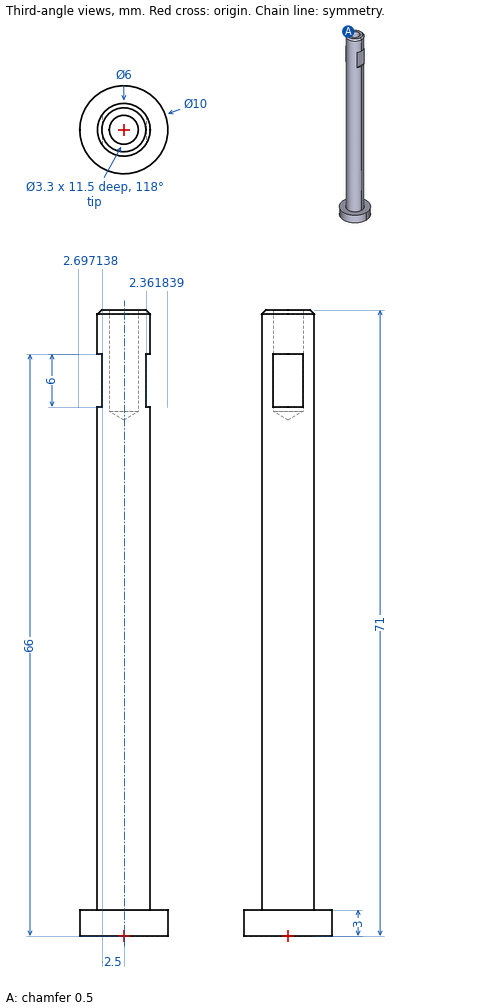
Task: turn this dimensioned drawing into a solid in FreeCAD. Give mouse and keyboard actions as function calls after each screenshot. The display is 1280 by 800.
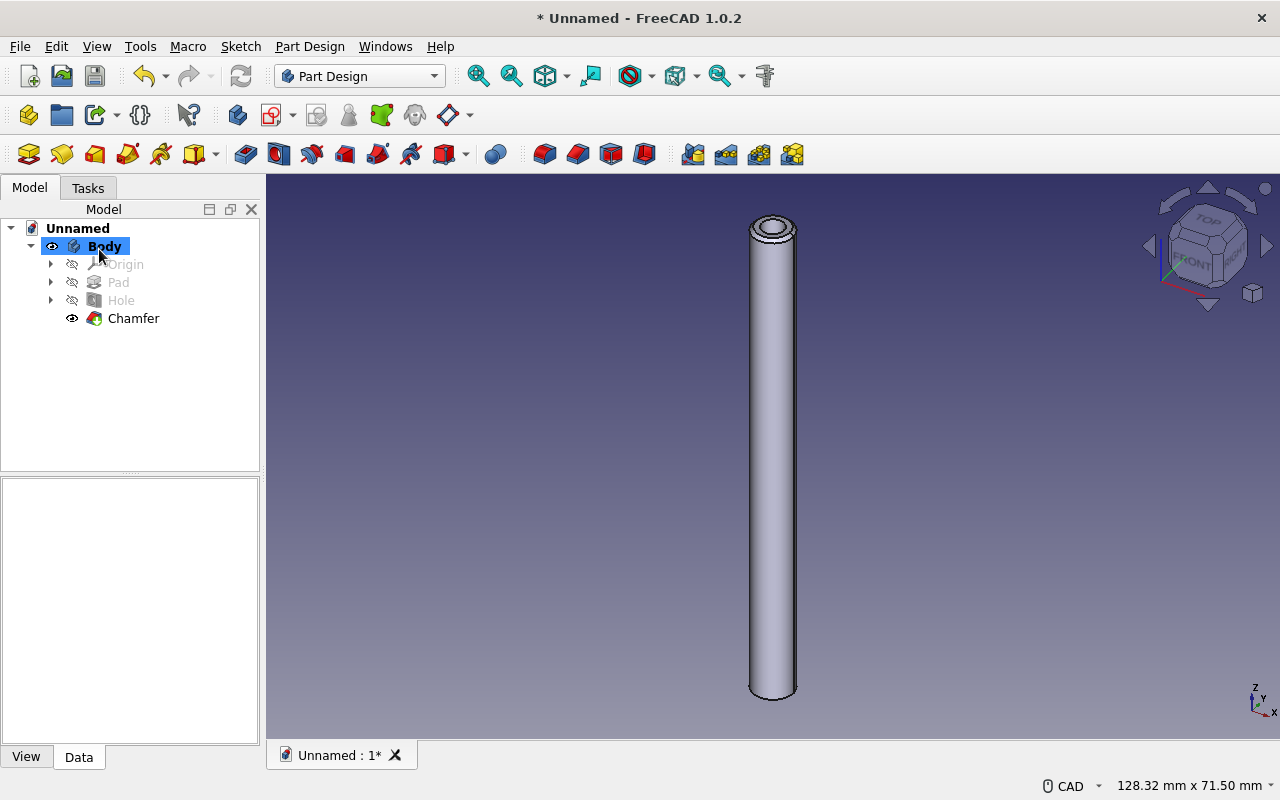
click(270, 116)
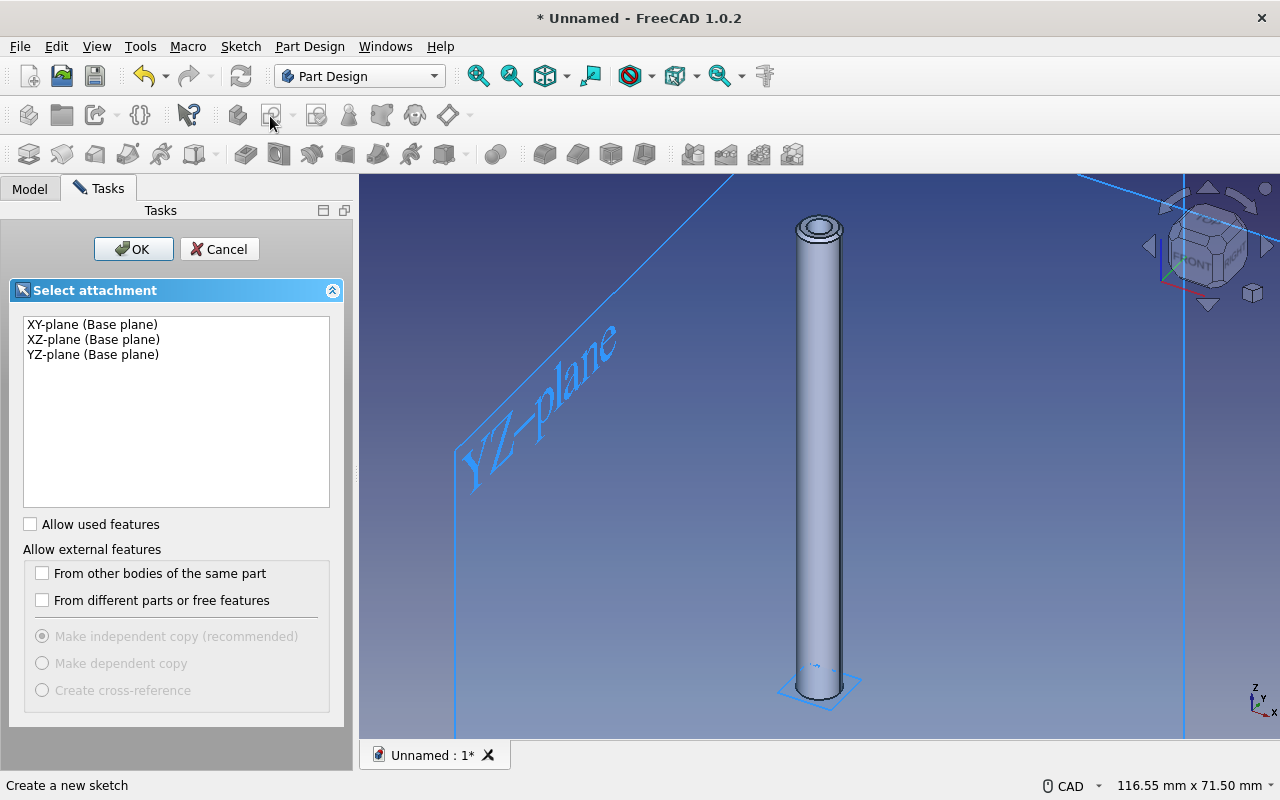
click(84, 340)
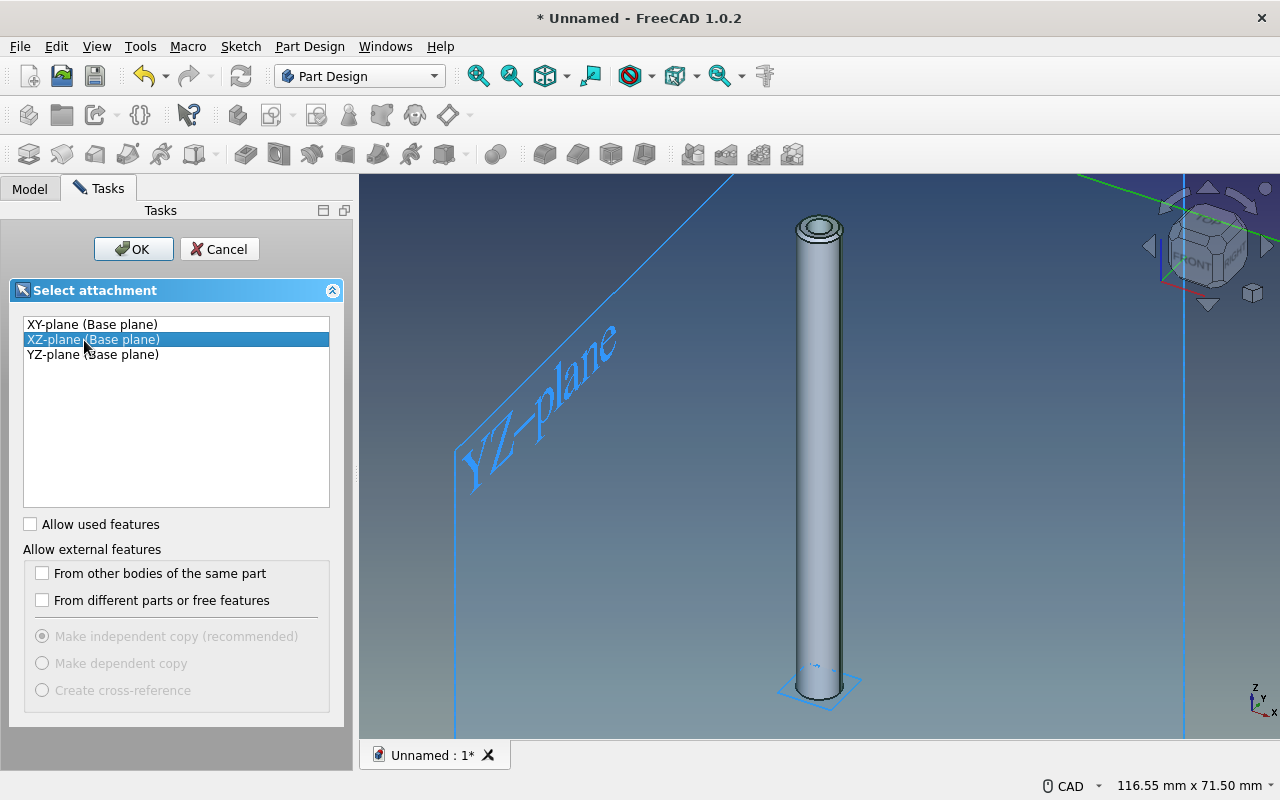
click(134, 249)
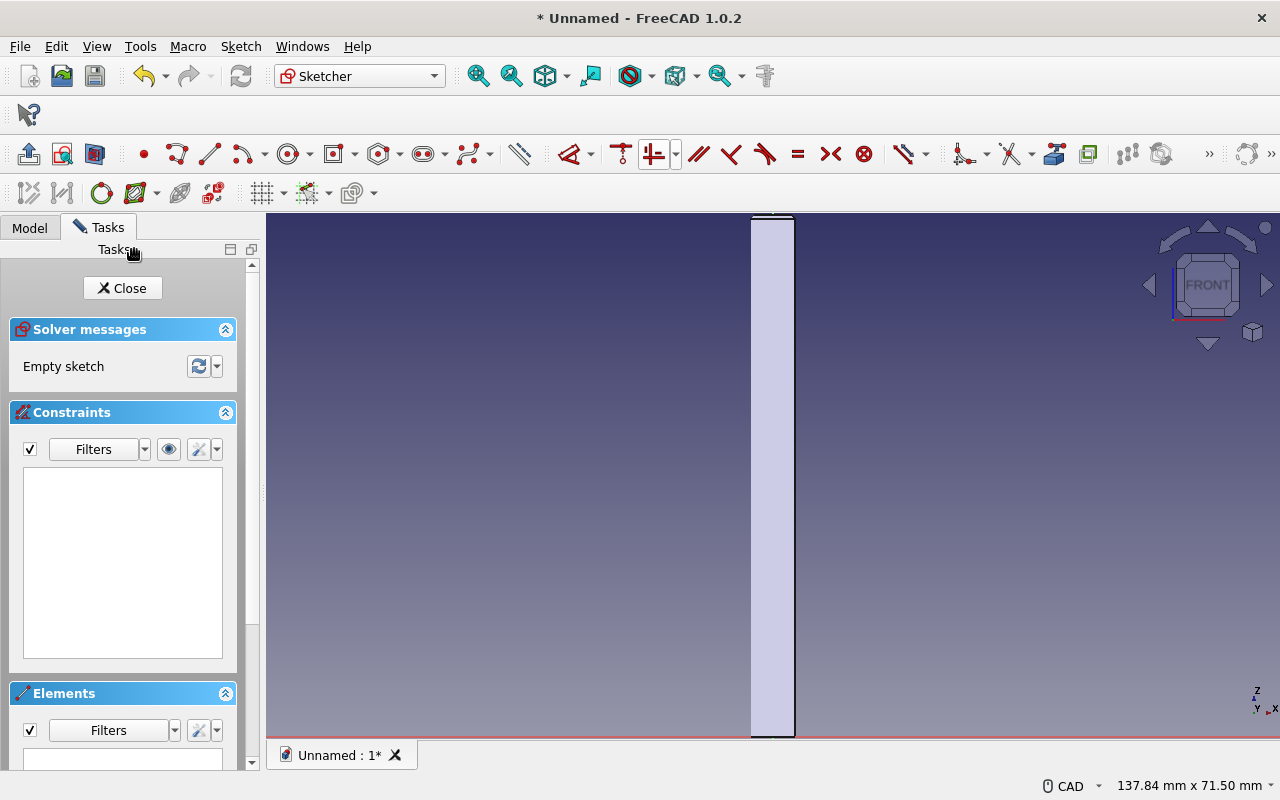
key(q)
key(s)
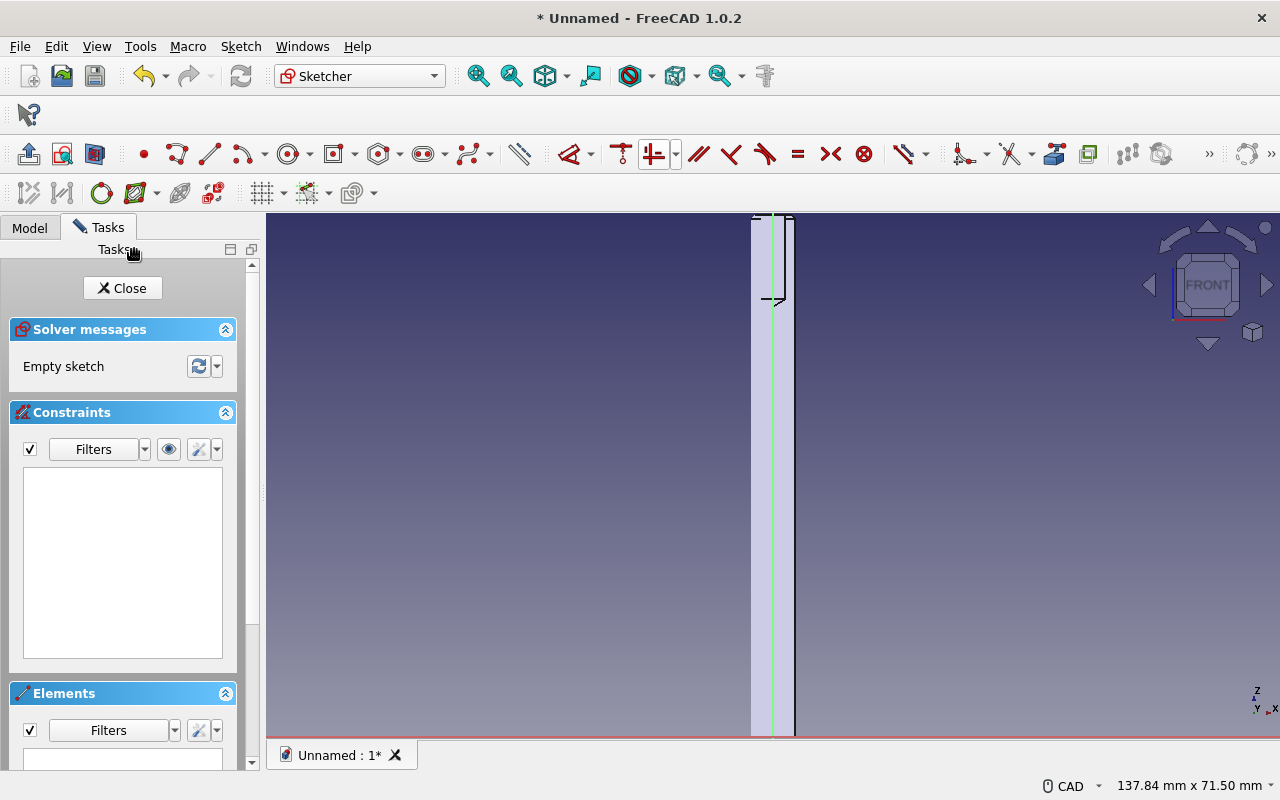
scroll(782, 242, up, 10)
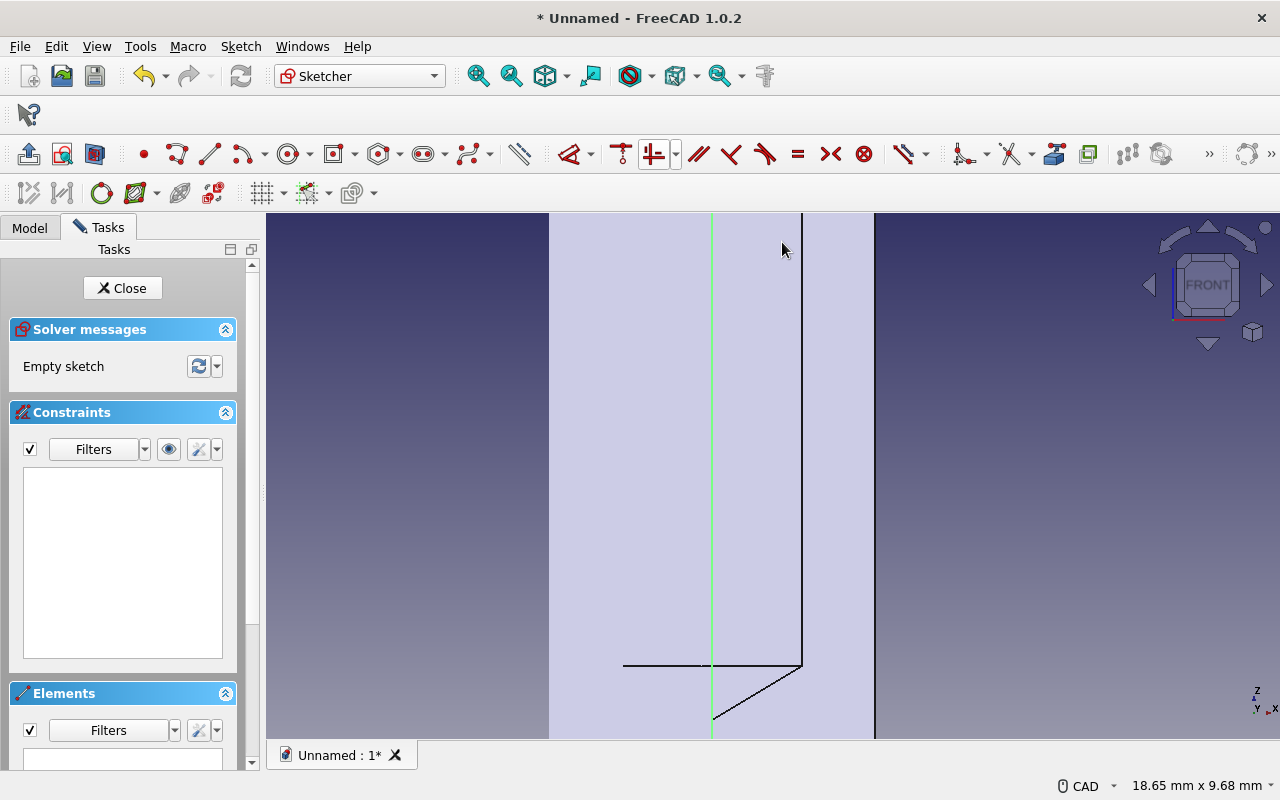
key(g)
key(r)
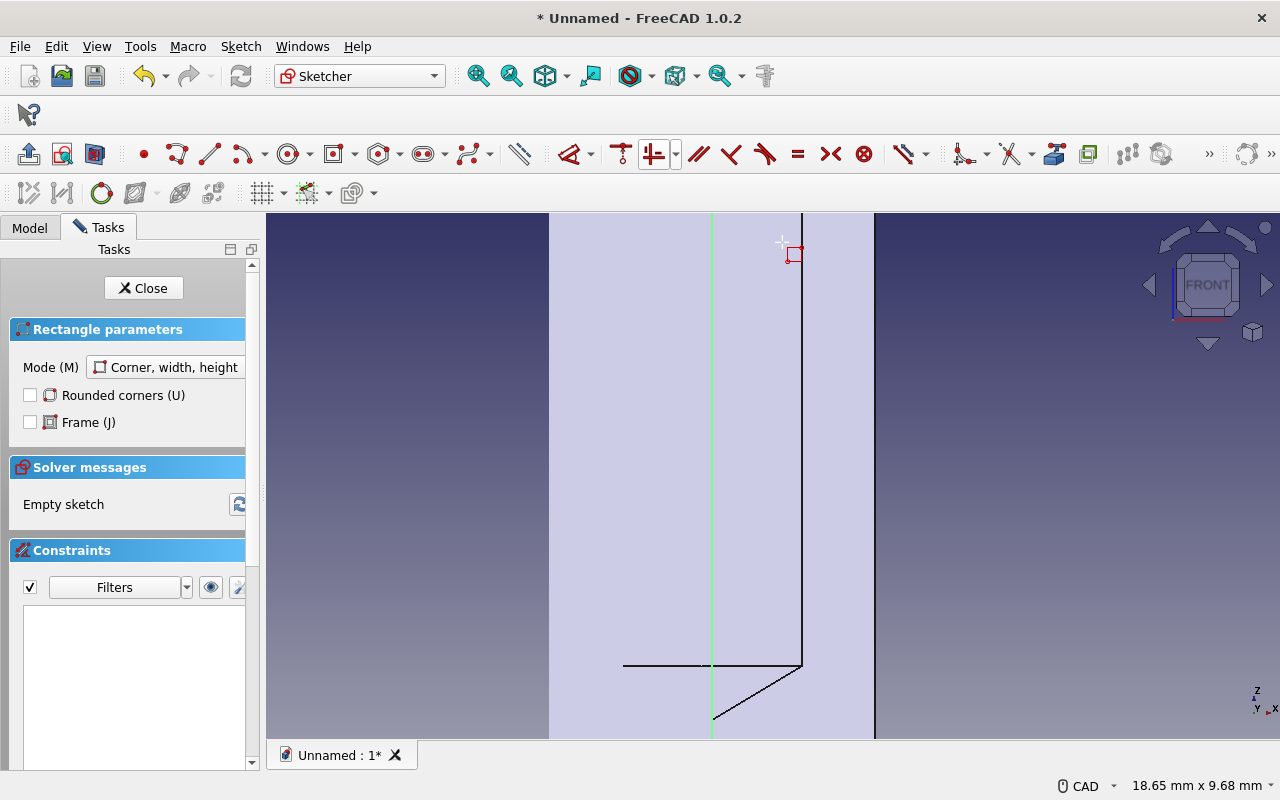
click(430, 313)
move(576, 639)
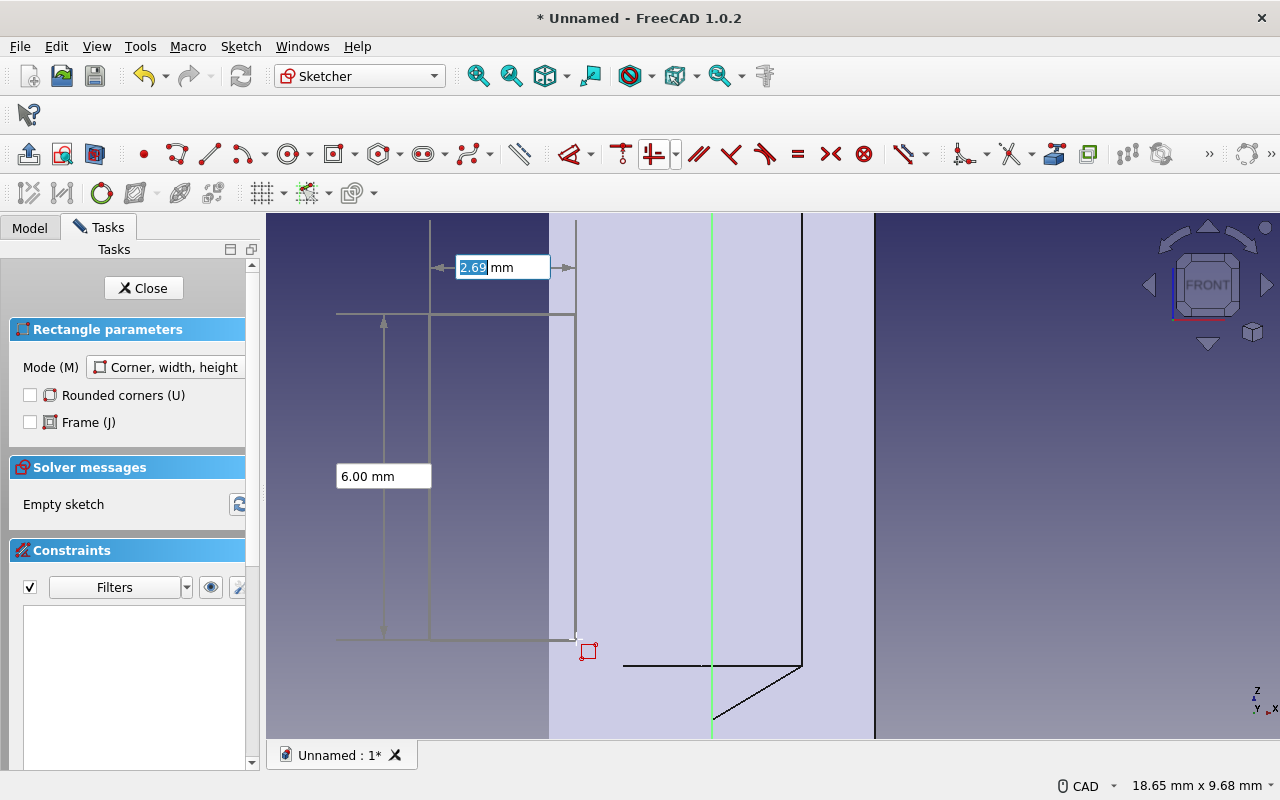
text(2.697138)
key(Tab)
text(6)
key(Return)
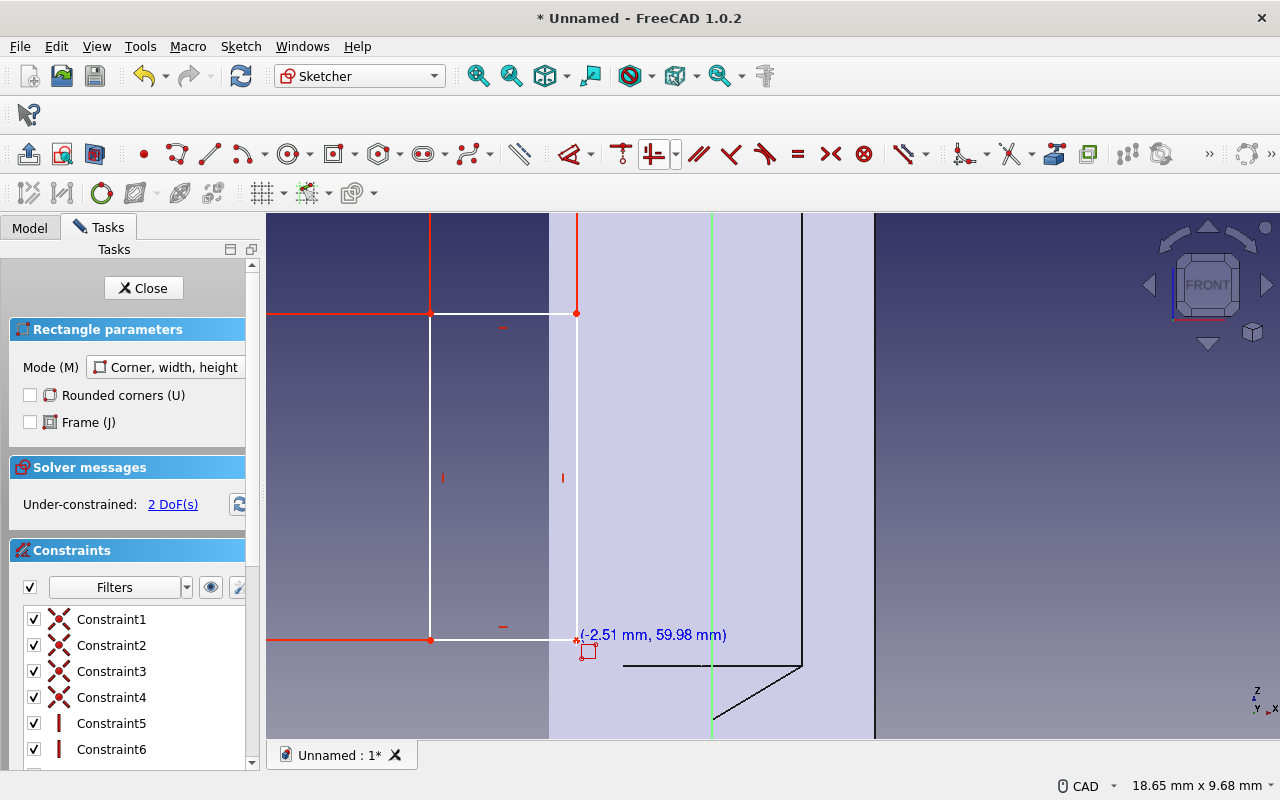
click(848, 313)
move(977, 639)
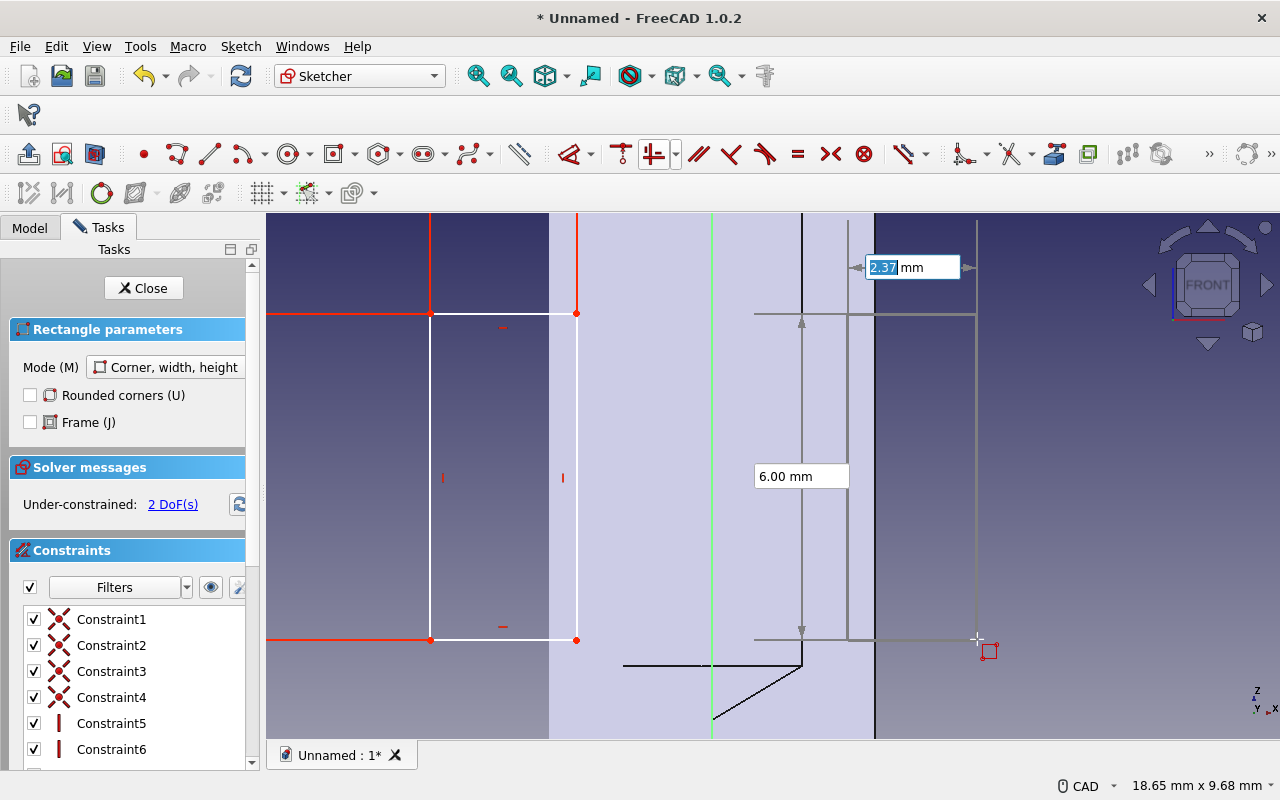
text(2.361839)
key(Tab)
text(6)
key(Return)
key(Escape)